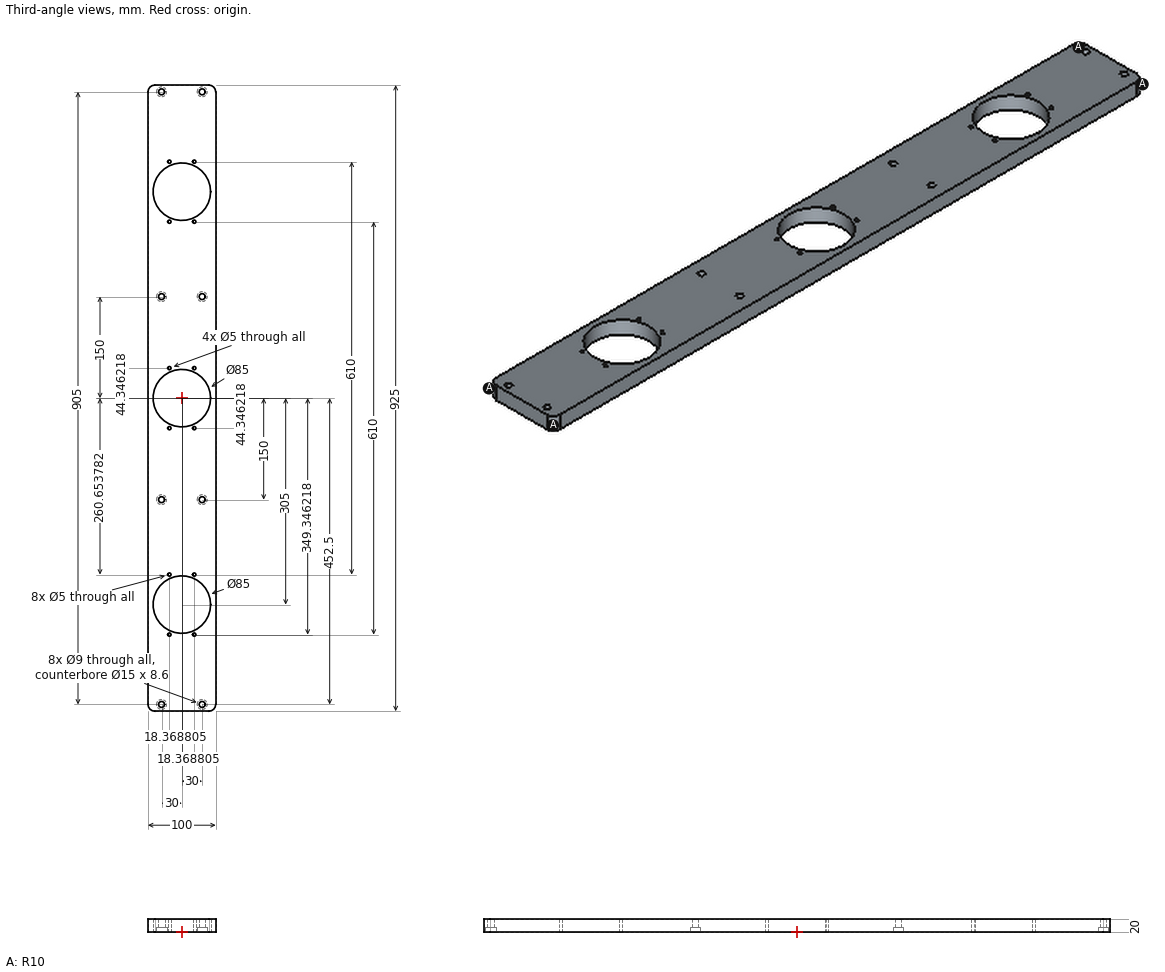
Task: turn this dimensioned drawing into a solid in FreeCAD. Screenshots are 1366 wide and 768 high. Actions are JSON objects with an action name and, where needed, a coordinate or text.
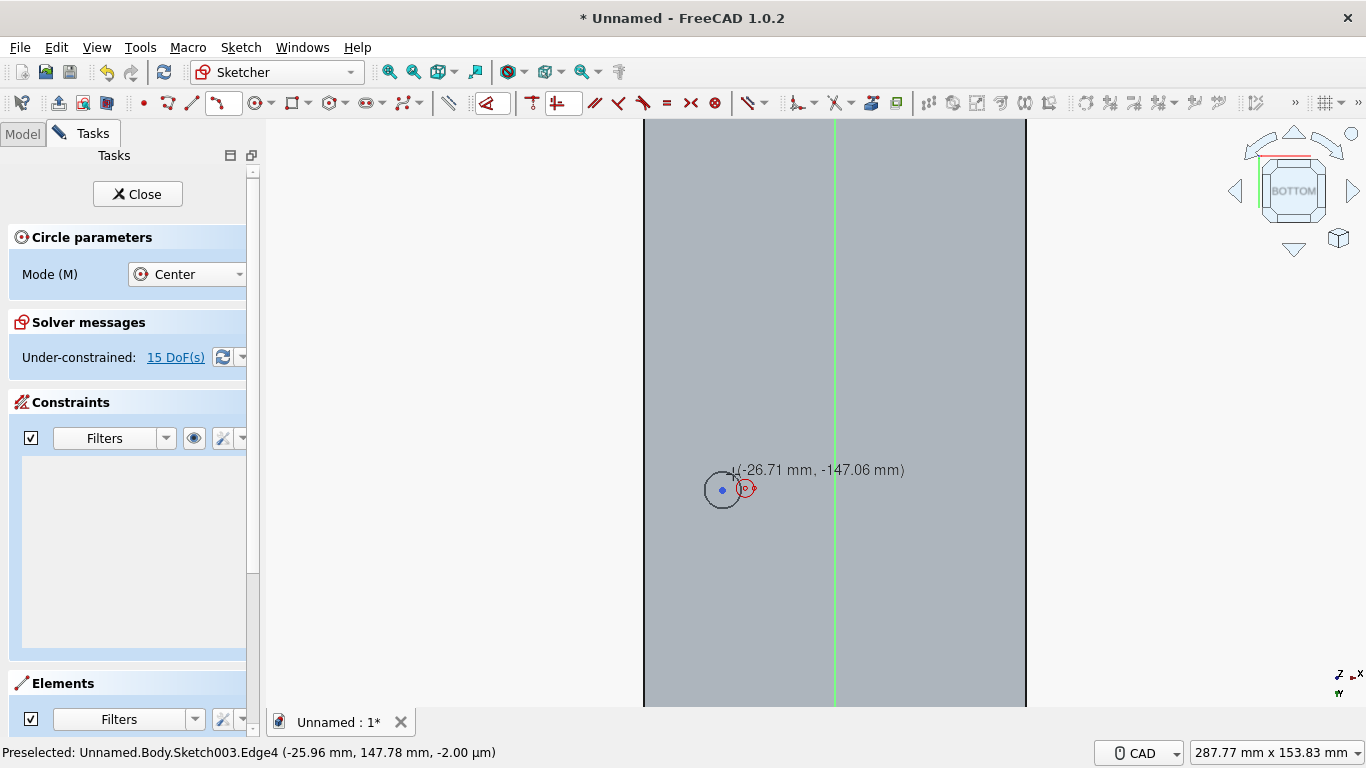
{"action": "scroll", "coordinate": [950, 486], "scroll_direction": "up", "scroll_amount": 2}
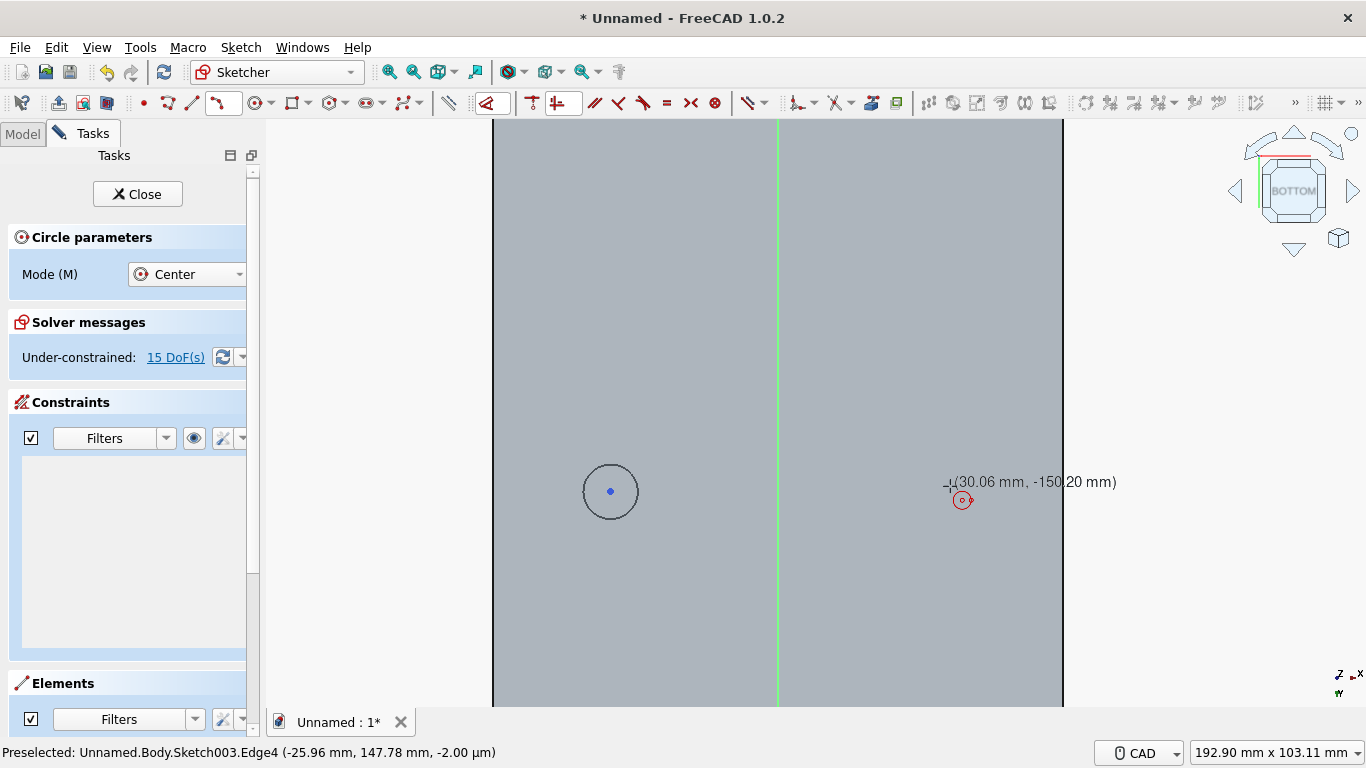
{"action": "scroll", "coordinate": [745, 476], "scroll_direction": "down", "scroll_amount": 13}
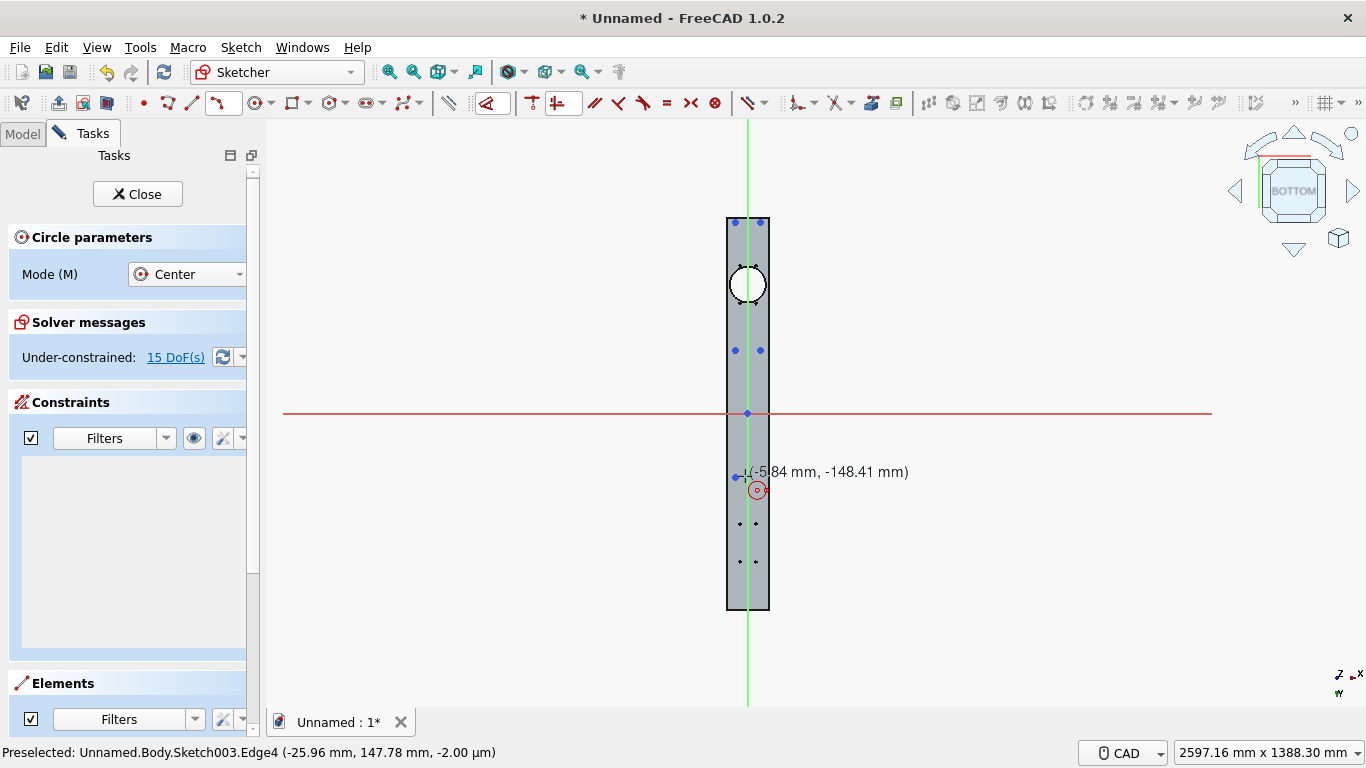
{"action": "scroll", "coordinate": [761, 477], "scroll_direction": "up", "scroll_amount": 2}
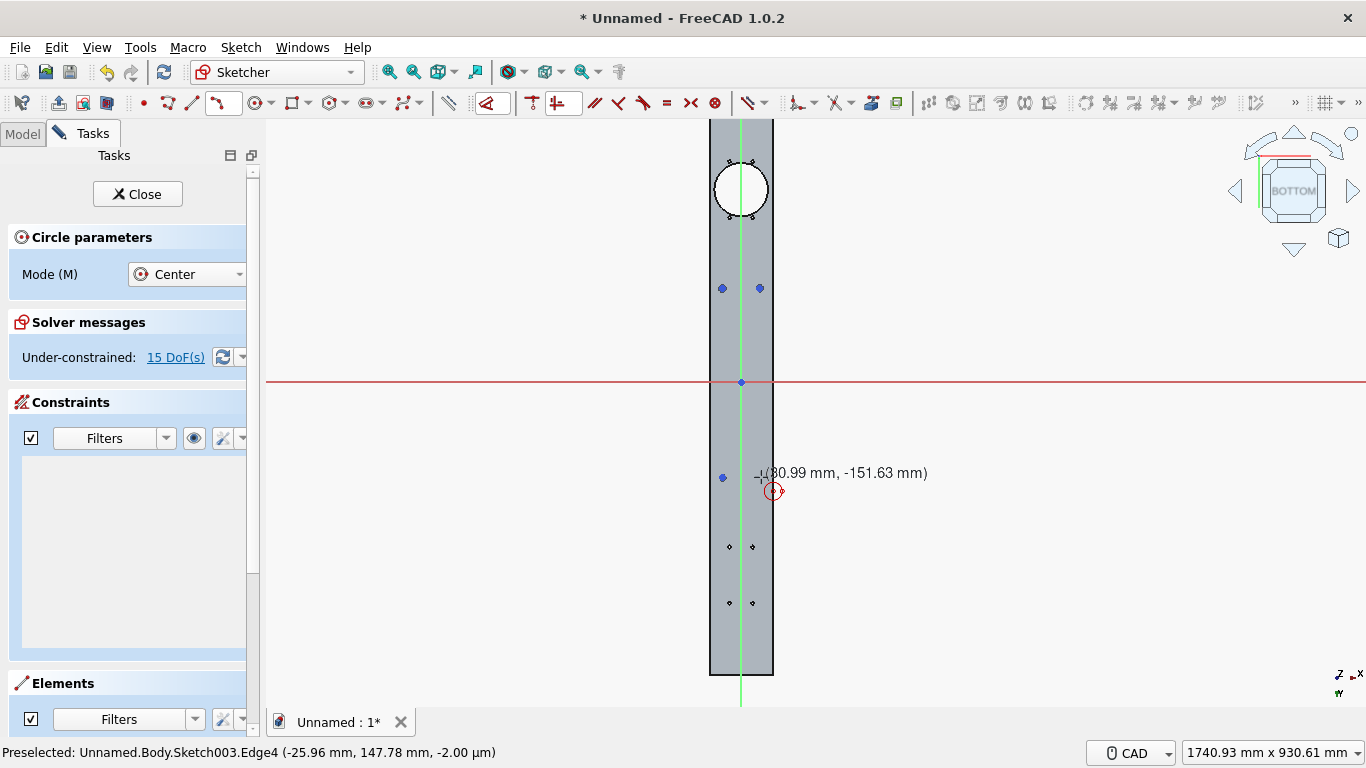
{"action": "left_click", "coordinate": [760, 477]}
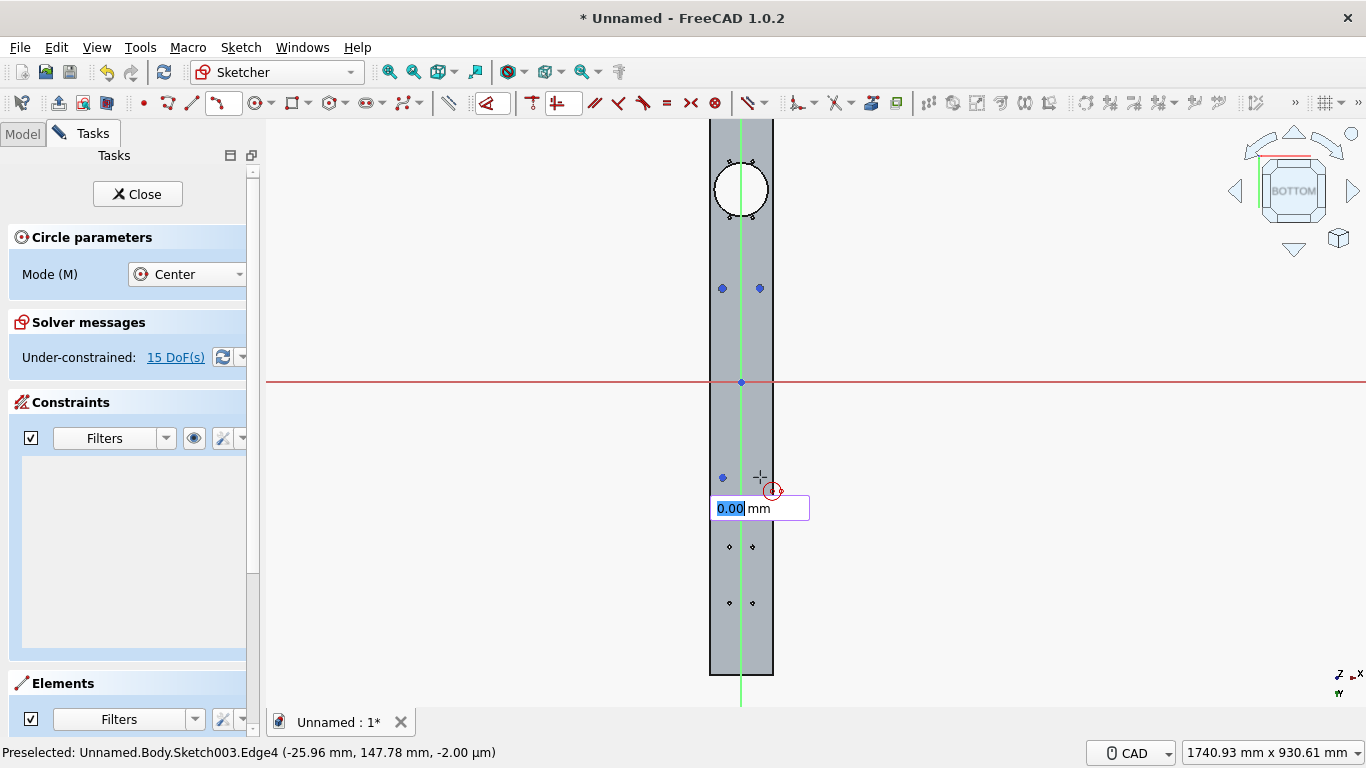
{"action": "scroll", "coordinate": [762, 475], "scroll_direction": "up", "scroll_amount": 9}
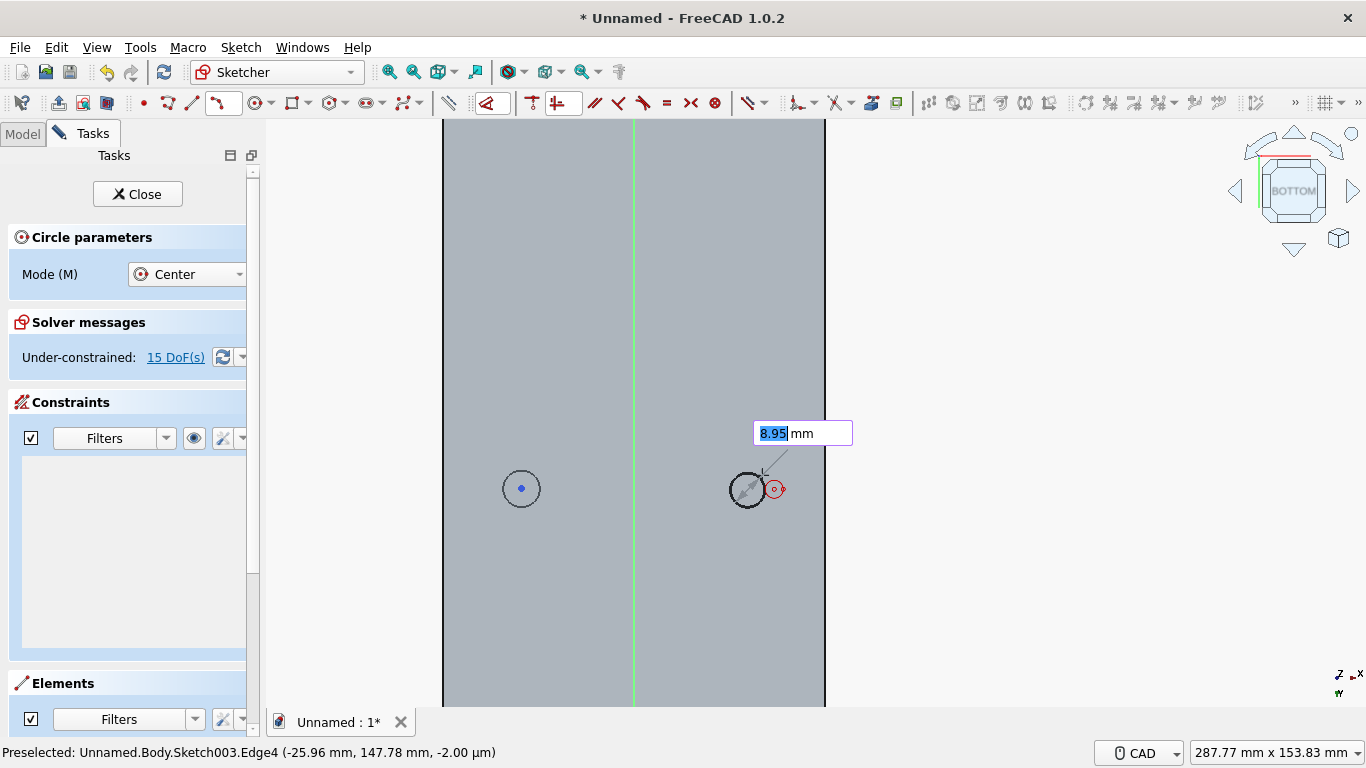
{"action": "left_click", "coordinate": [761, 473]}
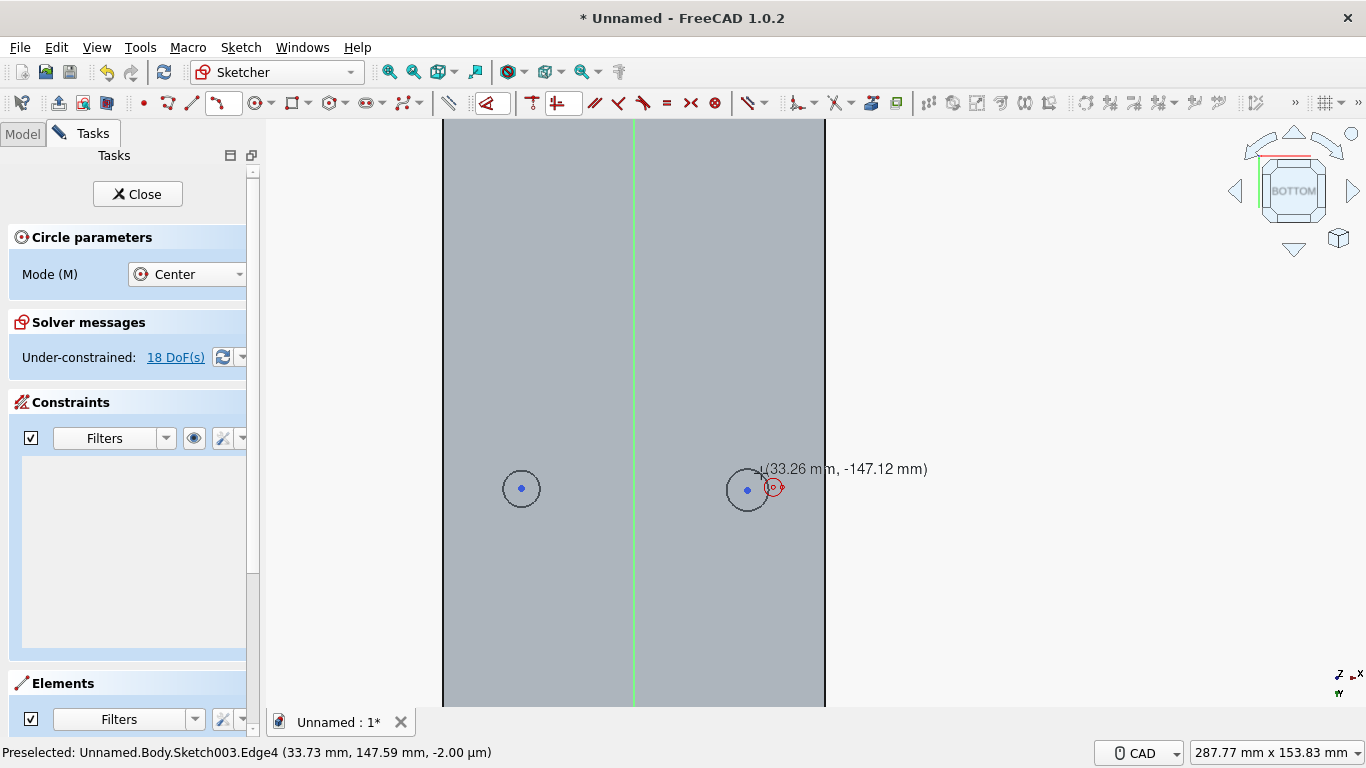
{"action": "scroll", "coordinate": [762, 475], "scroll_direction": "down", "scroll_amount": 11}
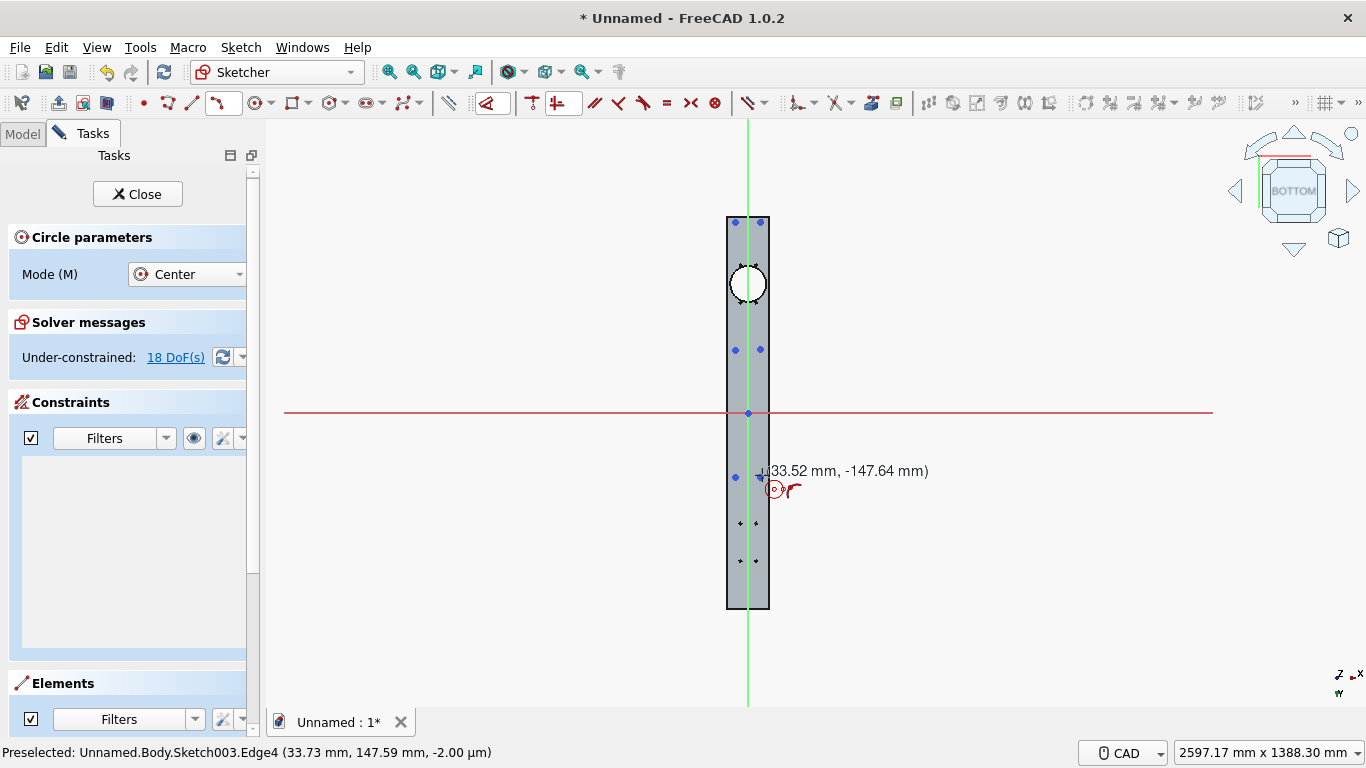
{"action": "scroll", "coordinate": [735, 605], "scroll_direction": "up", "scroll_amount": 13}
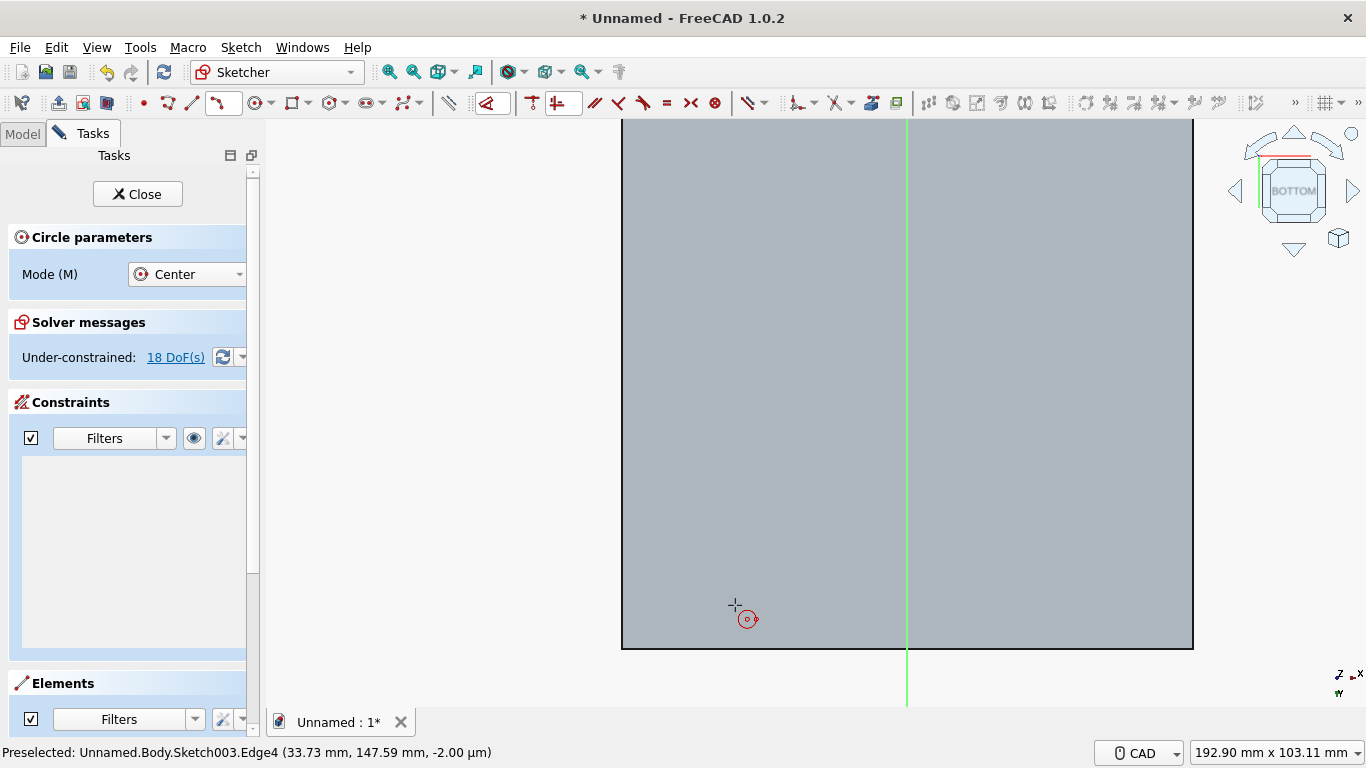
{"action": "scroll", "coordinate": [735, 606], "scroll_direction": "down", "scroll_amount": 13}